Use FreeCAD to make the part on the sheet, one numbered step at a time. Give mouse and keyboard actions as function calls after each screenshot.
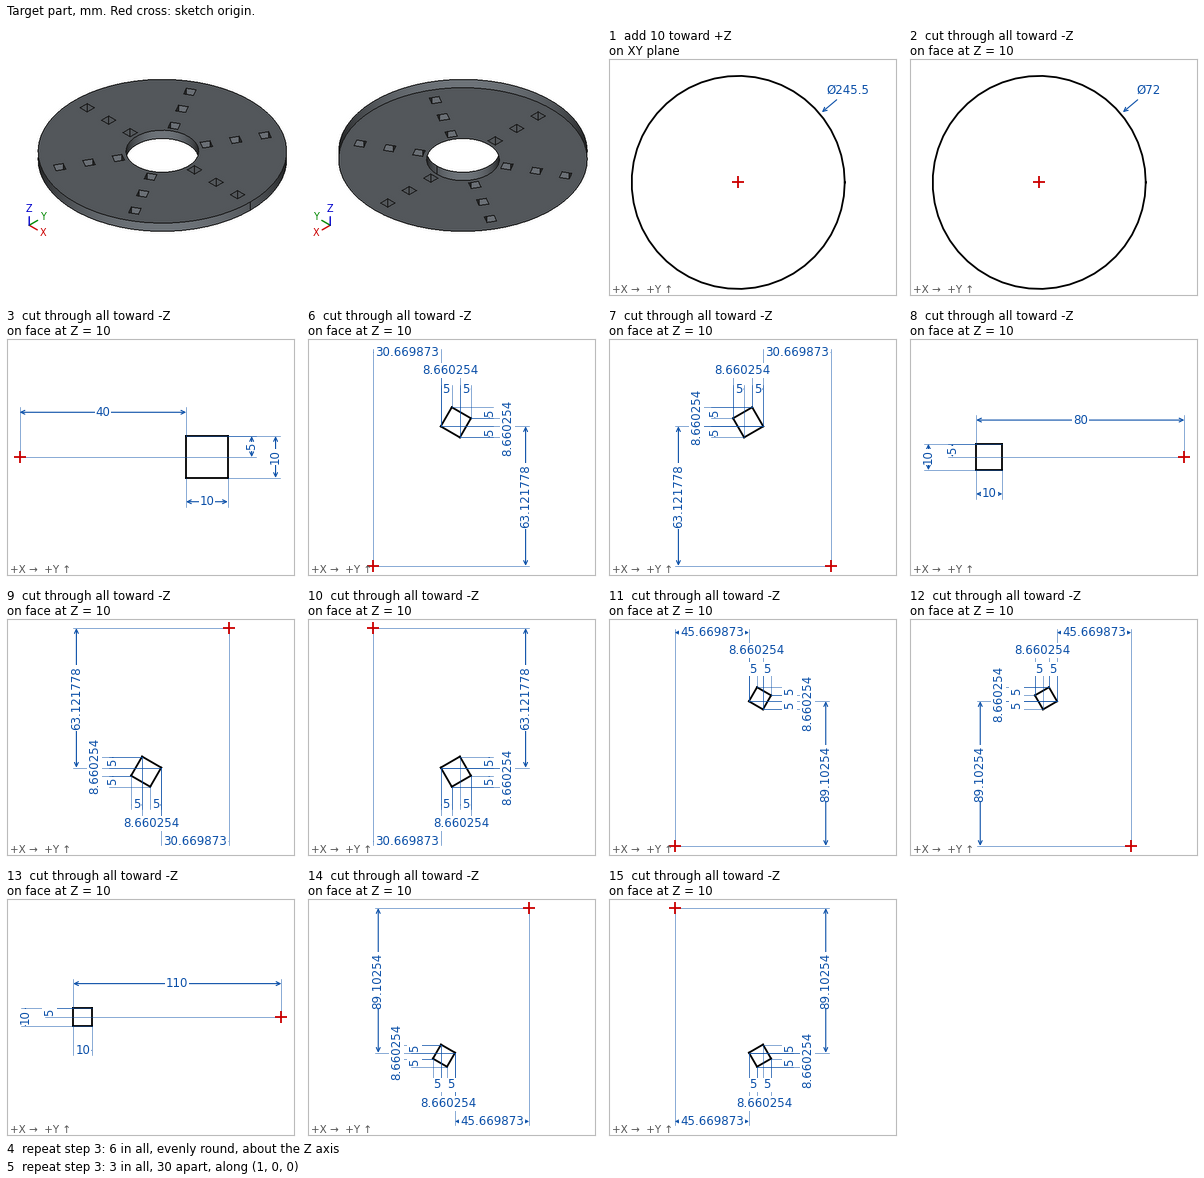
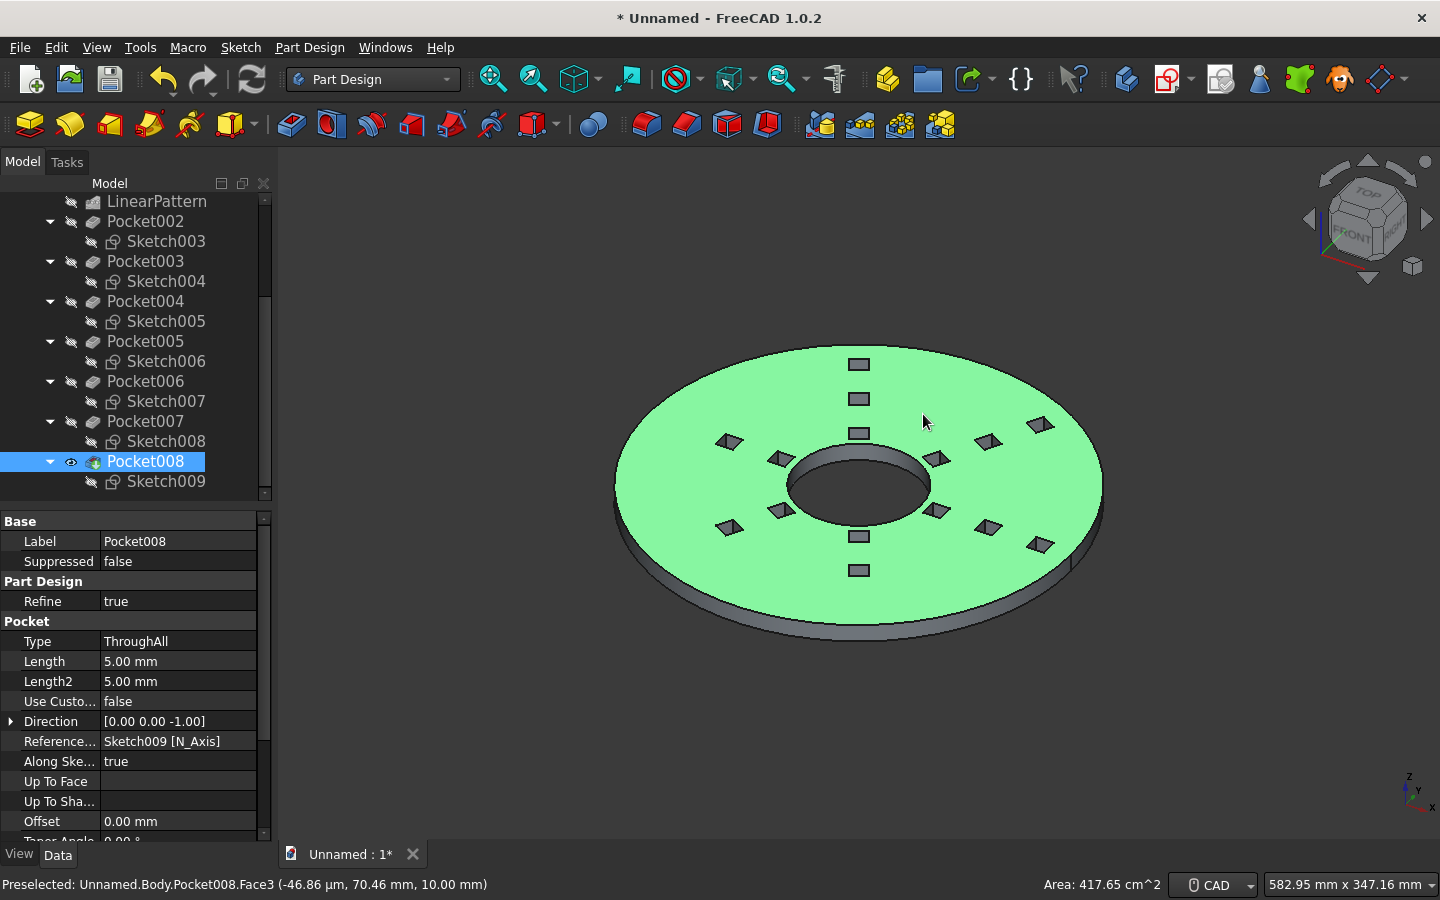
click(1168, 80)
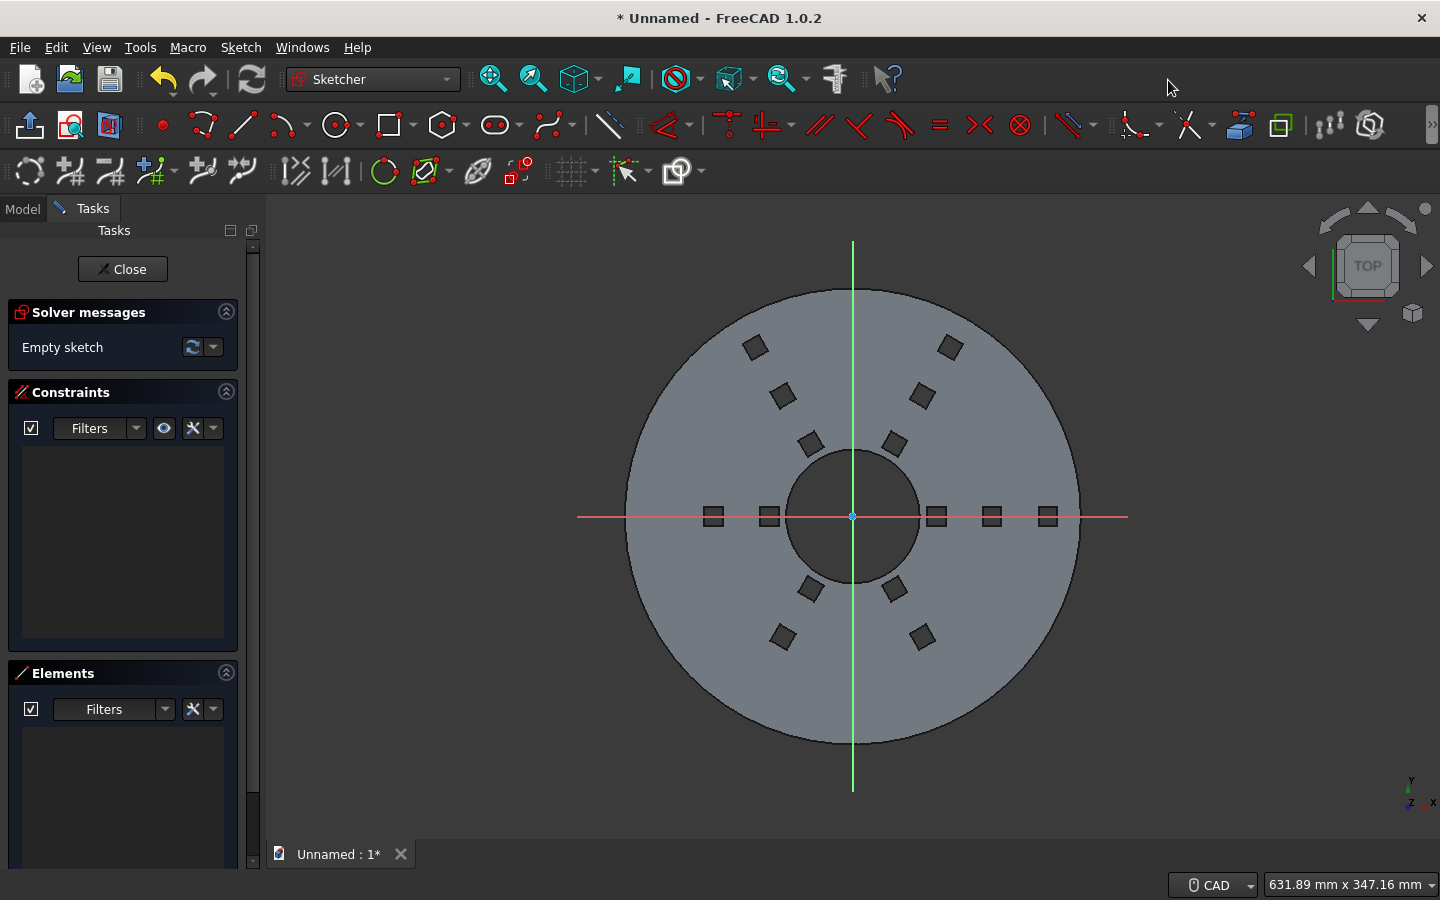
scroll(651, 517, up, 15)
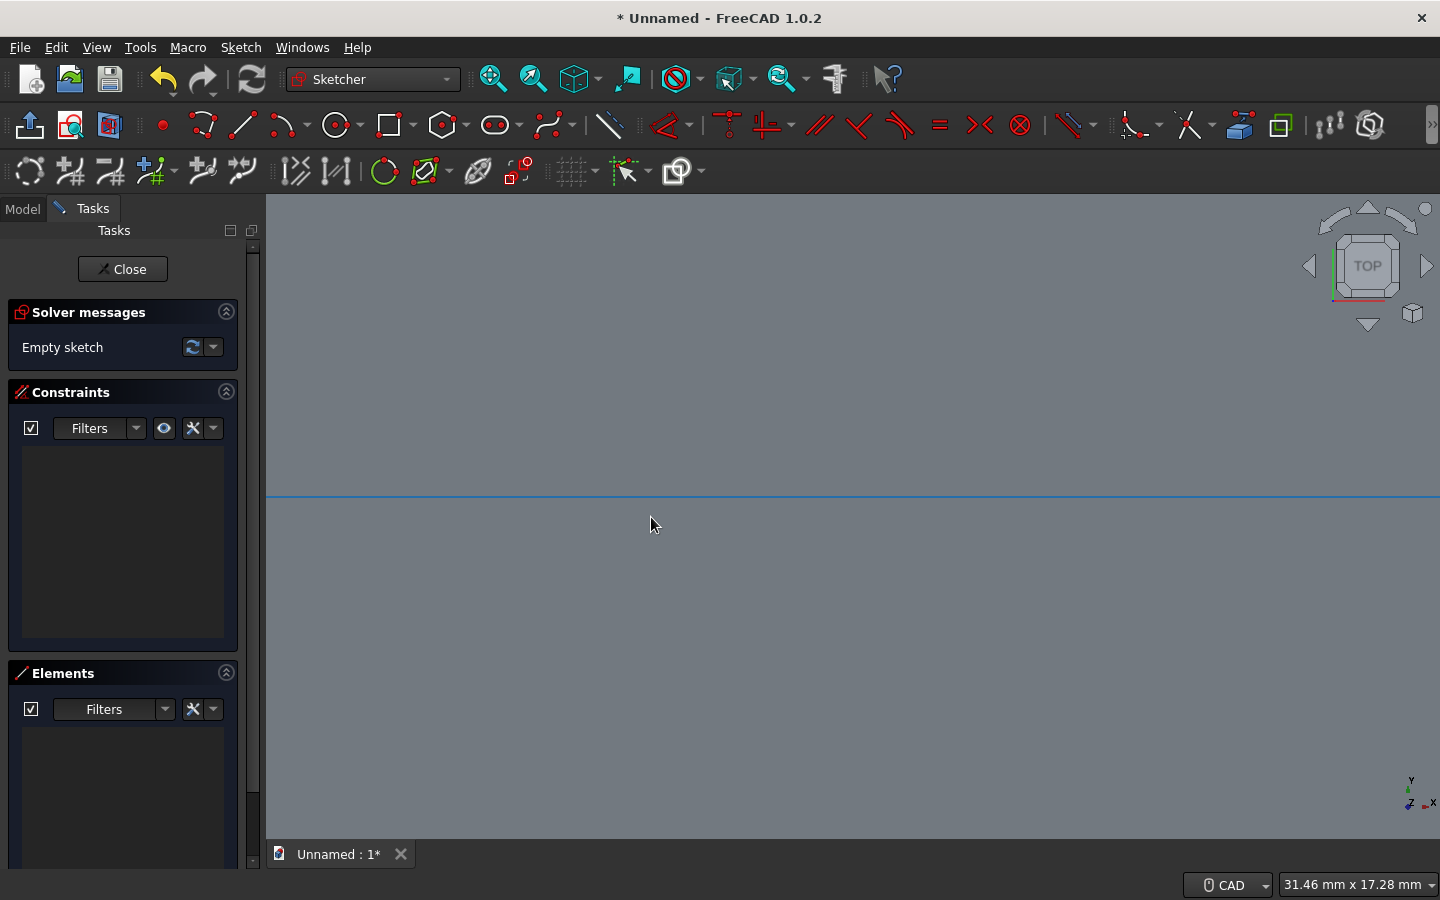
key(g)
key(r)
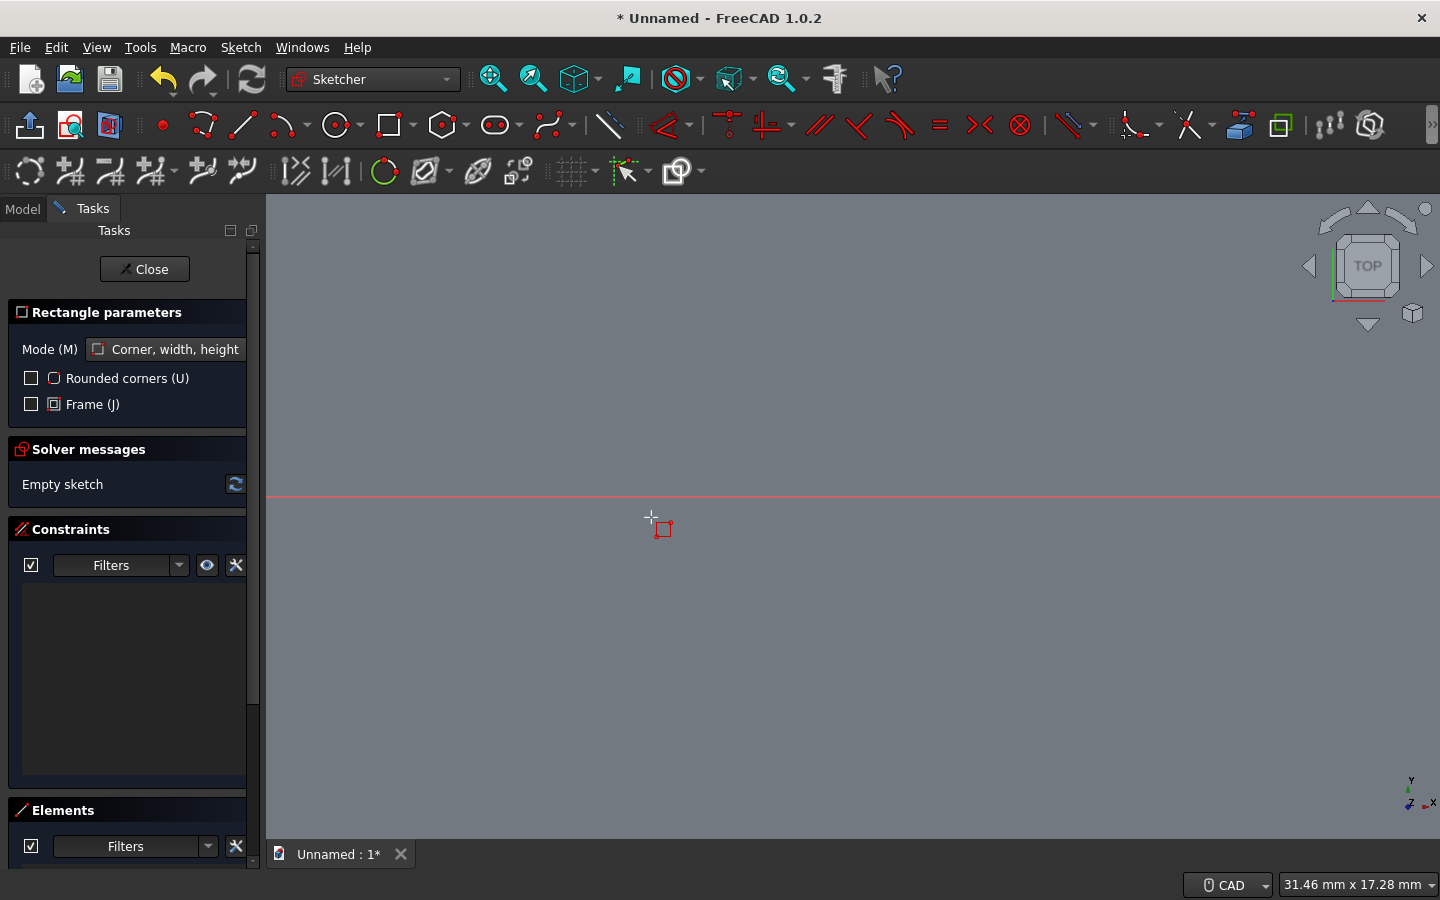
click(594, 311)
move(967, 684)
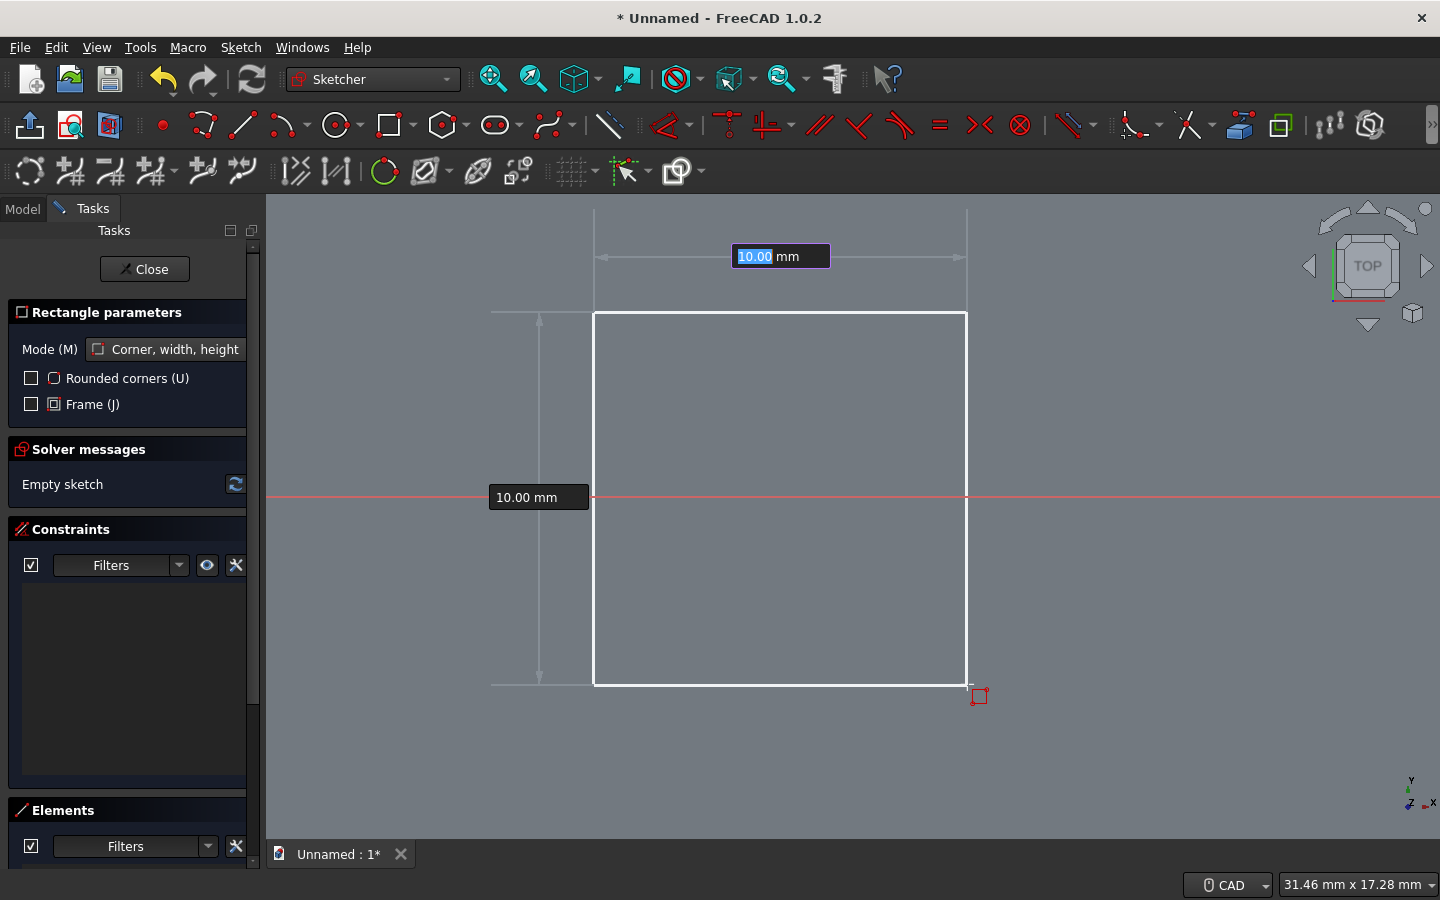
text(10)
key(Tab)
text(10)
key(Return)
key(Escape)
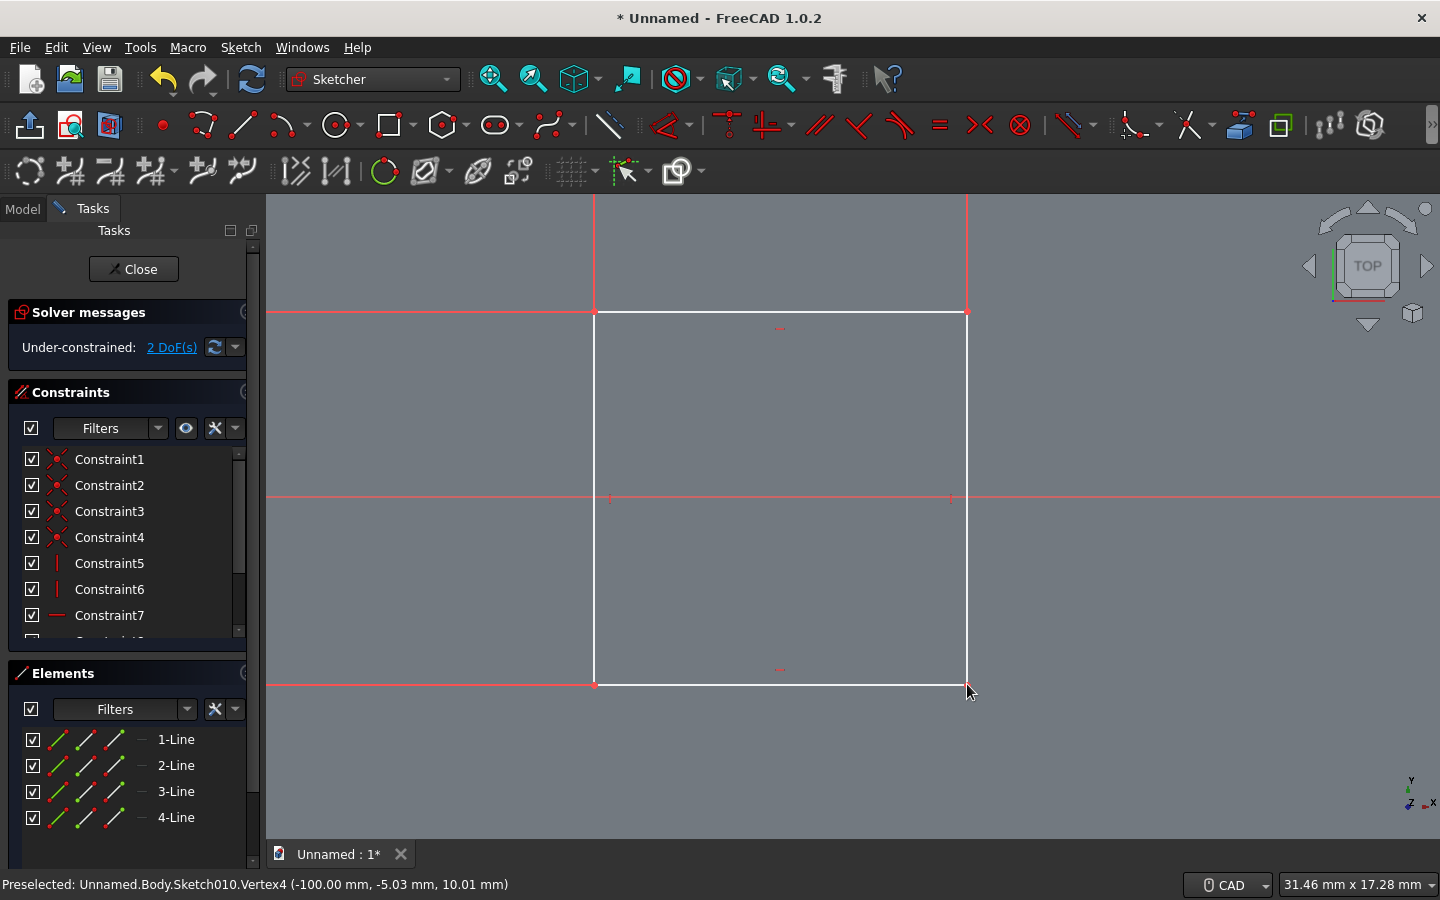
key(d)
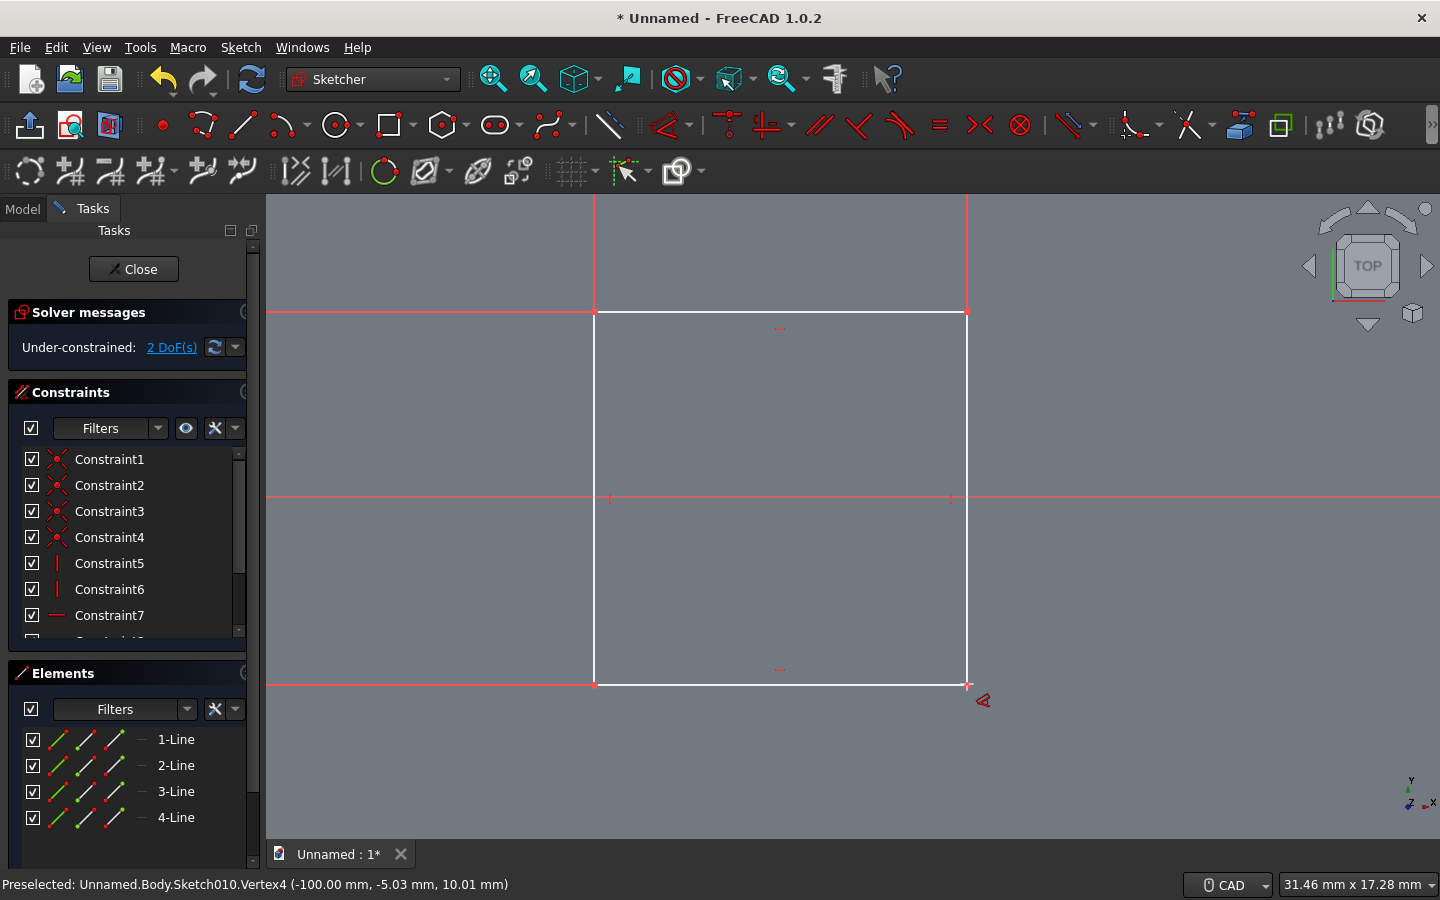
click(594, 312)
click(560, 405)